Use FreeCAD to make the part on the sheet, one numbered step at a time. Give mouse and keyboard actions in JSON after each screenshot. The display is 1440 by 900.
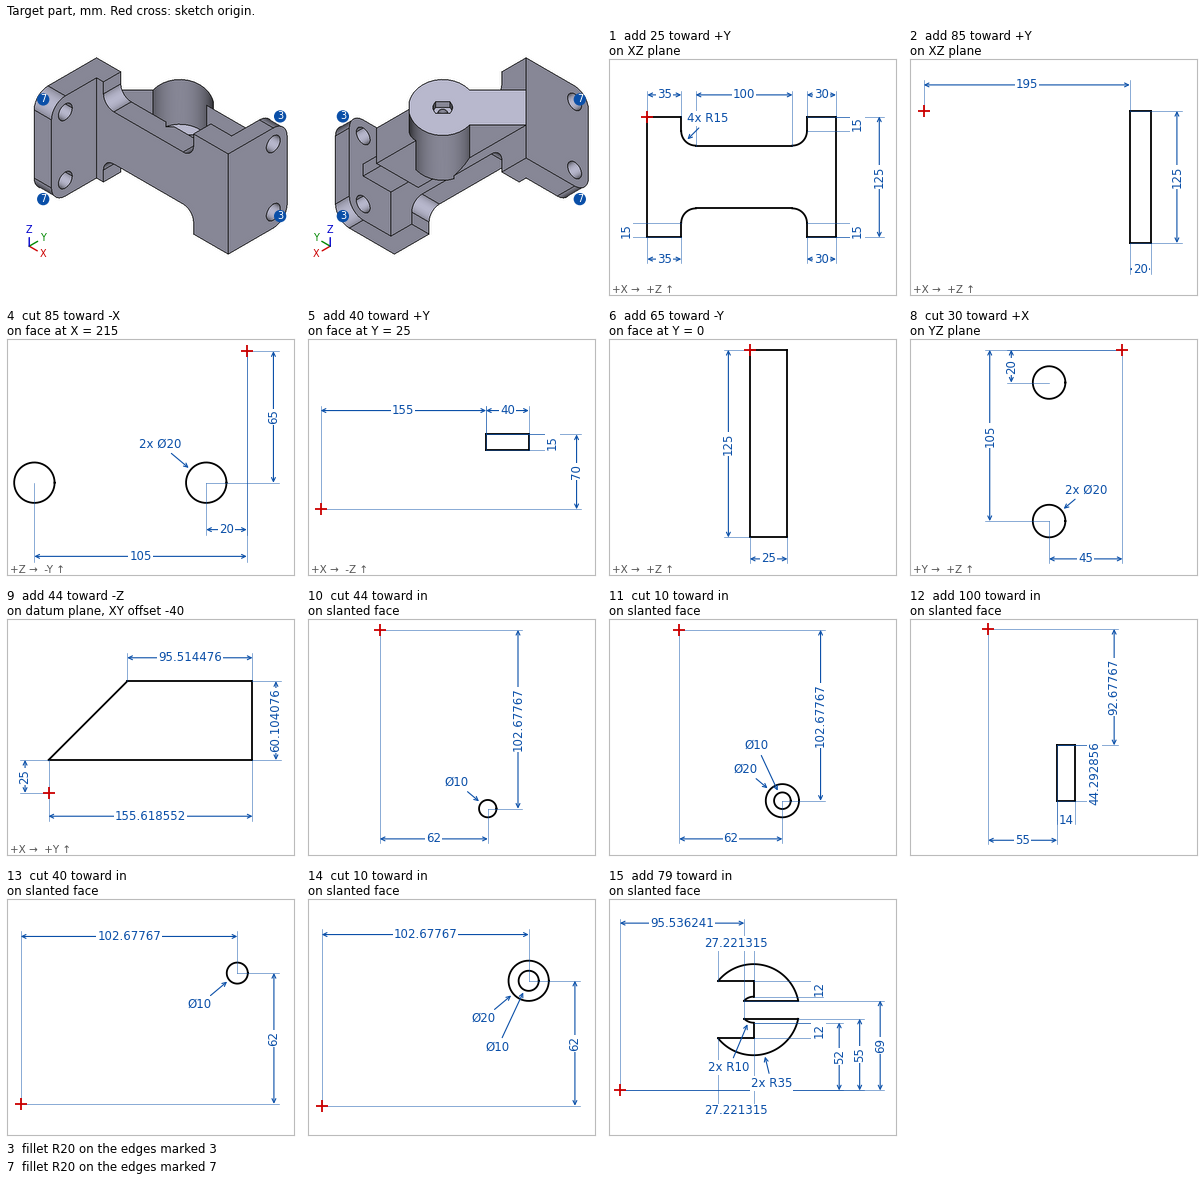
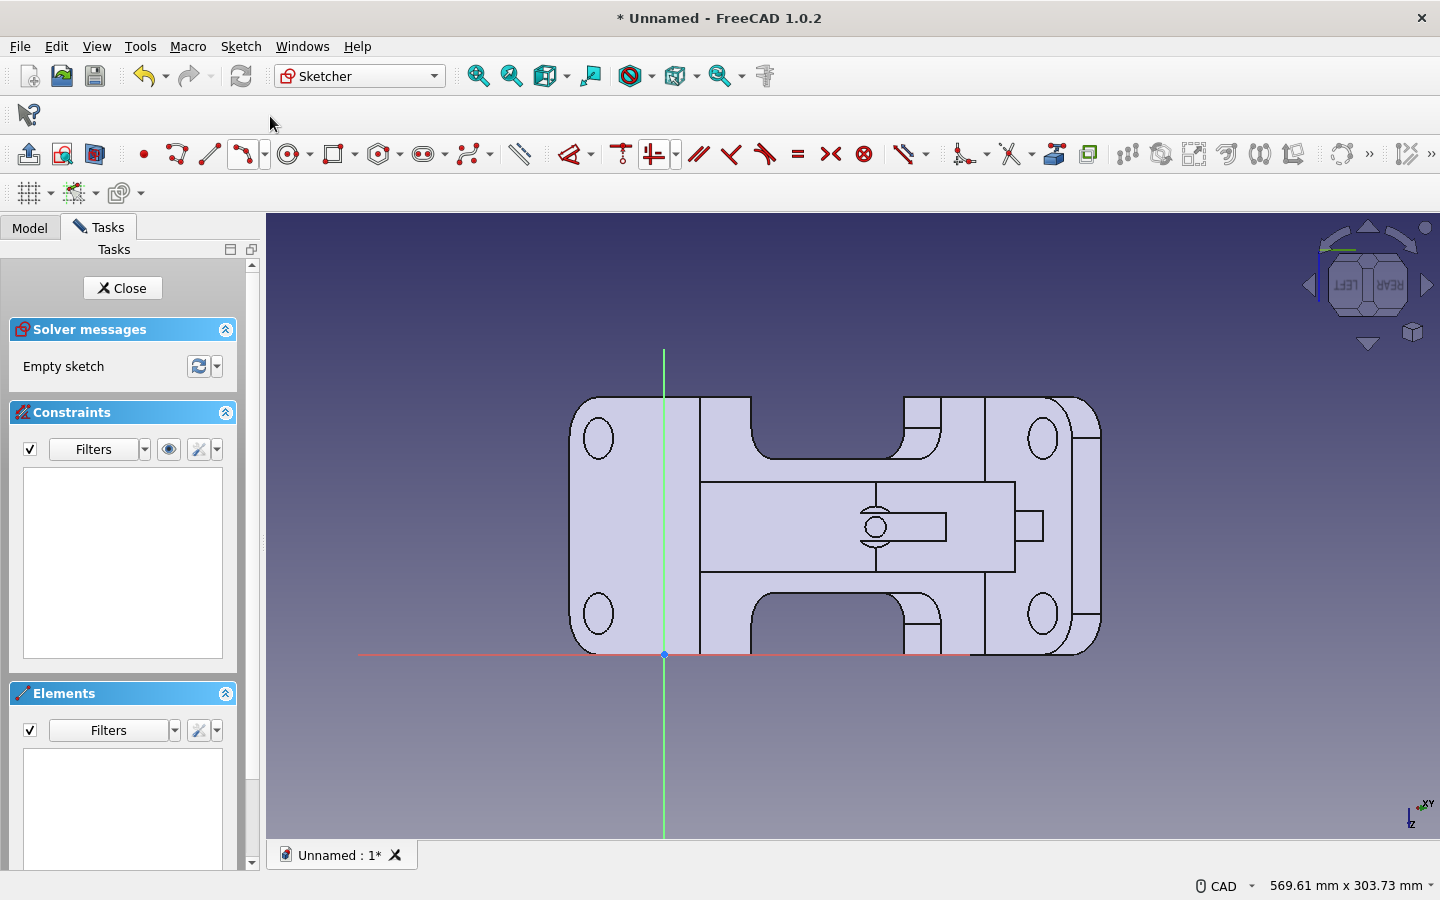
{"action": "scroll", "coordinate": [887, 527], "scroll_direction": "up", "scroll_amount": 11}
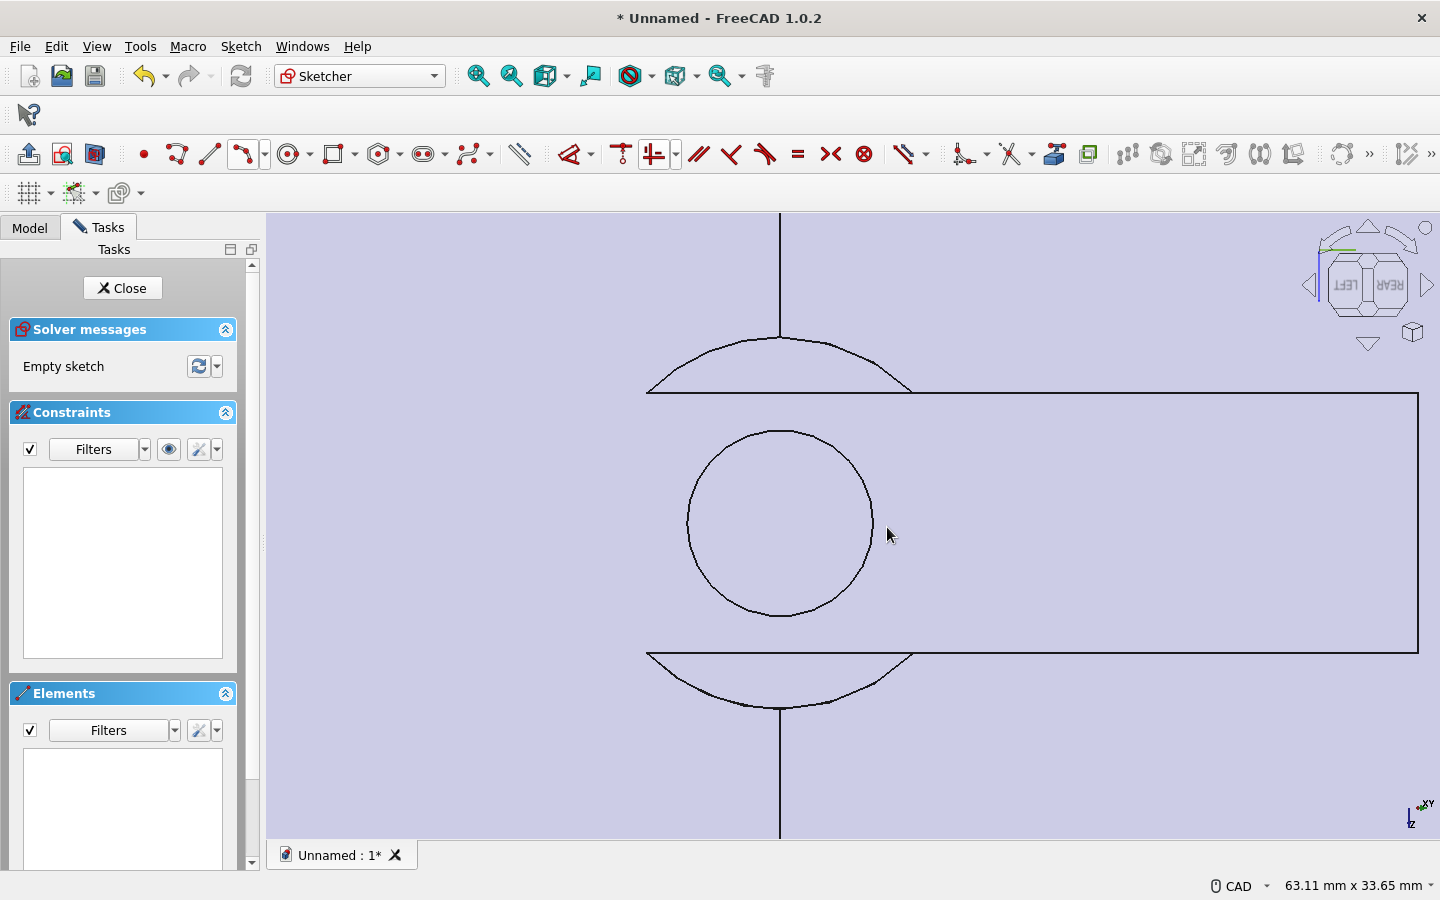
{"action": "key", "text": "g c"}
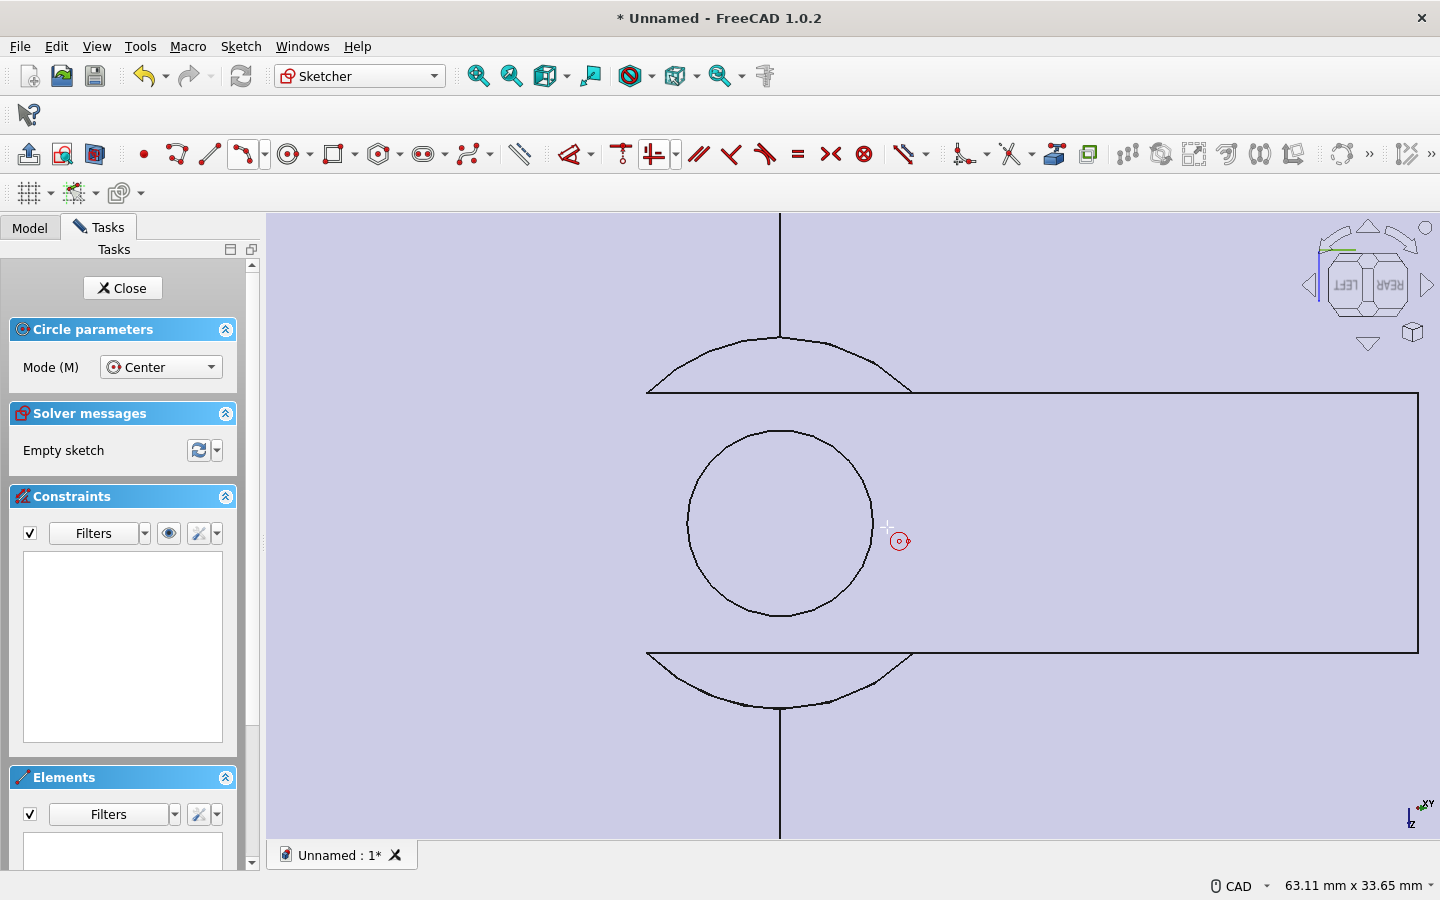
{"action": "left_click", "coordinate": [780, 523]}
{"action": "left_click", "coordinate": [912, 392]}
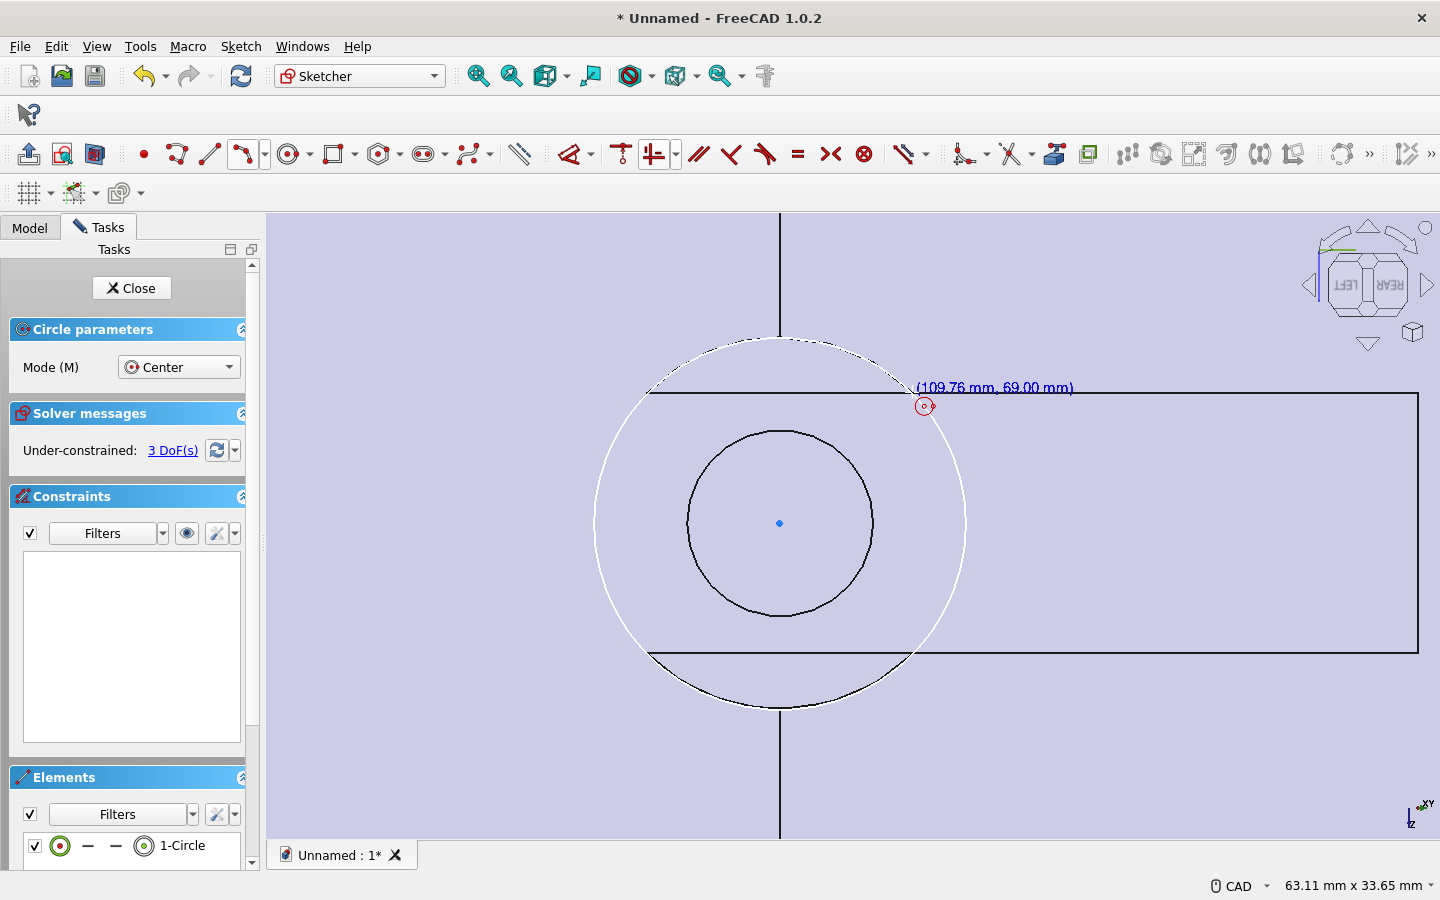
{"action": "left_click", "coordinate": [780, 524]}
{"action": "left_click", "coordinate": [846, 457]}
{"action": "key", "text": "Escape"}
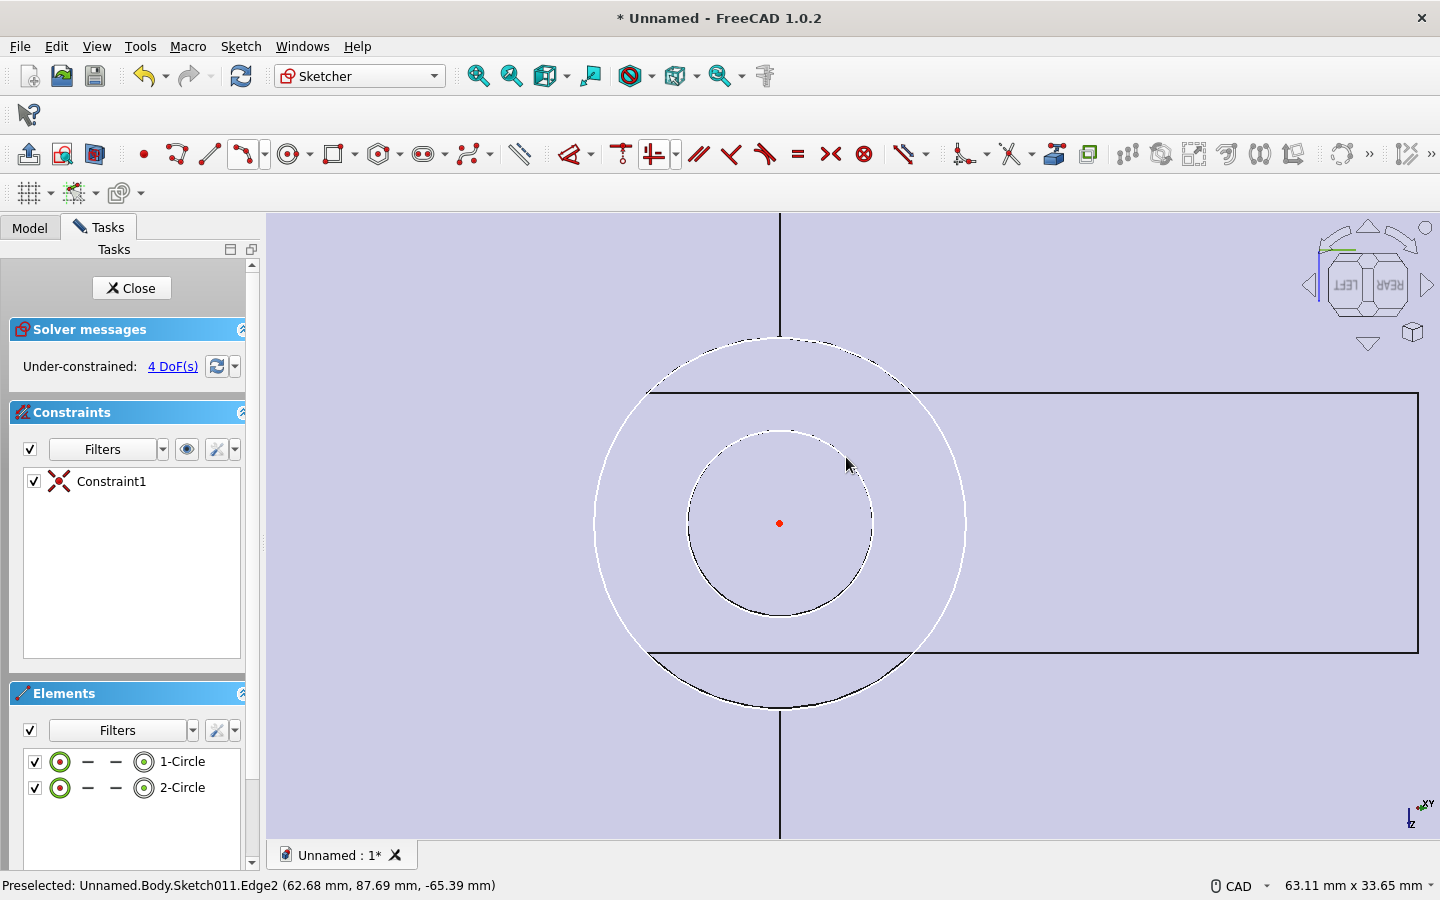
{"action": "left_click", "coordinate": [568, 154]}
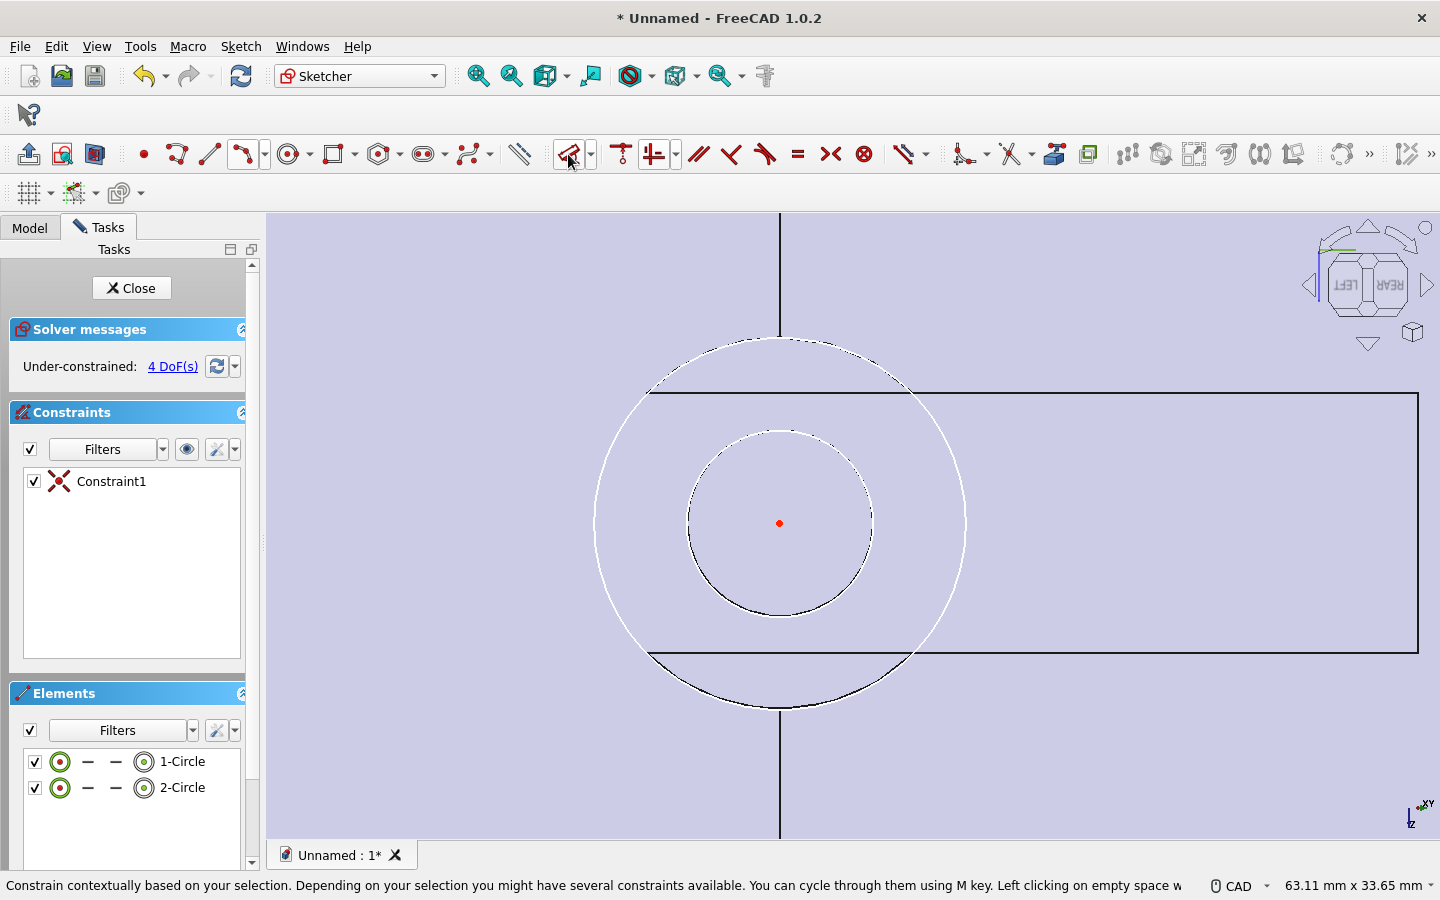
{"action": "left_click", "coordinate": [911, 392]}
{"action": "left_click", "coordinate": [934, 369]}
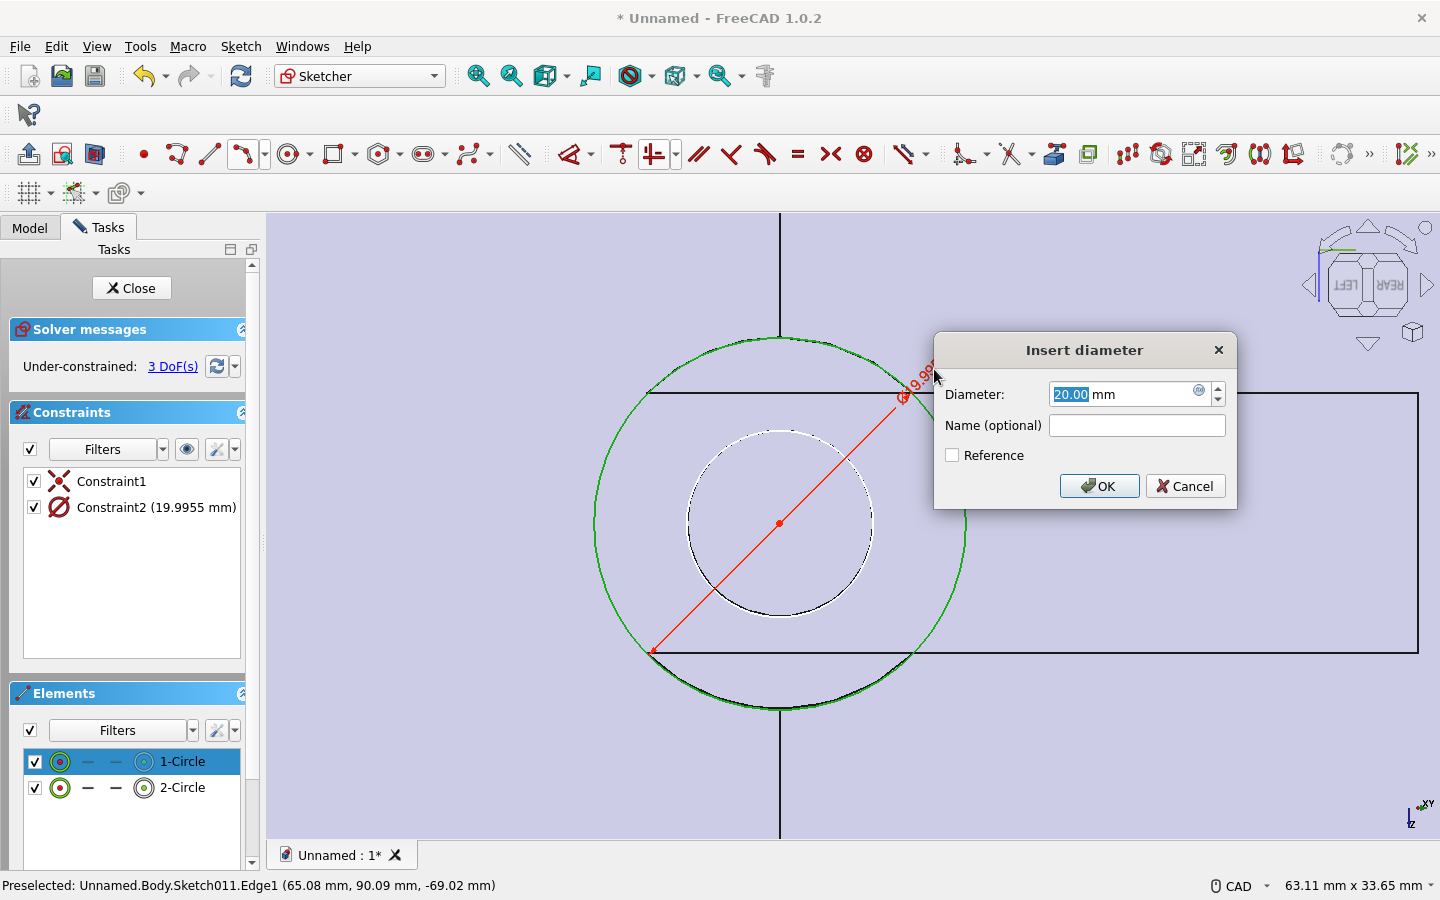
{"action": "type", "text": "20"}
{"action": "key", "text": "Return"}